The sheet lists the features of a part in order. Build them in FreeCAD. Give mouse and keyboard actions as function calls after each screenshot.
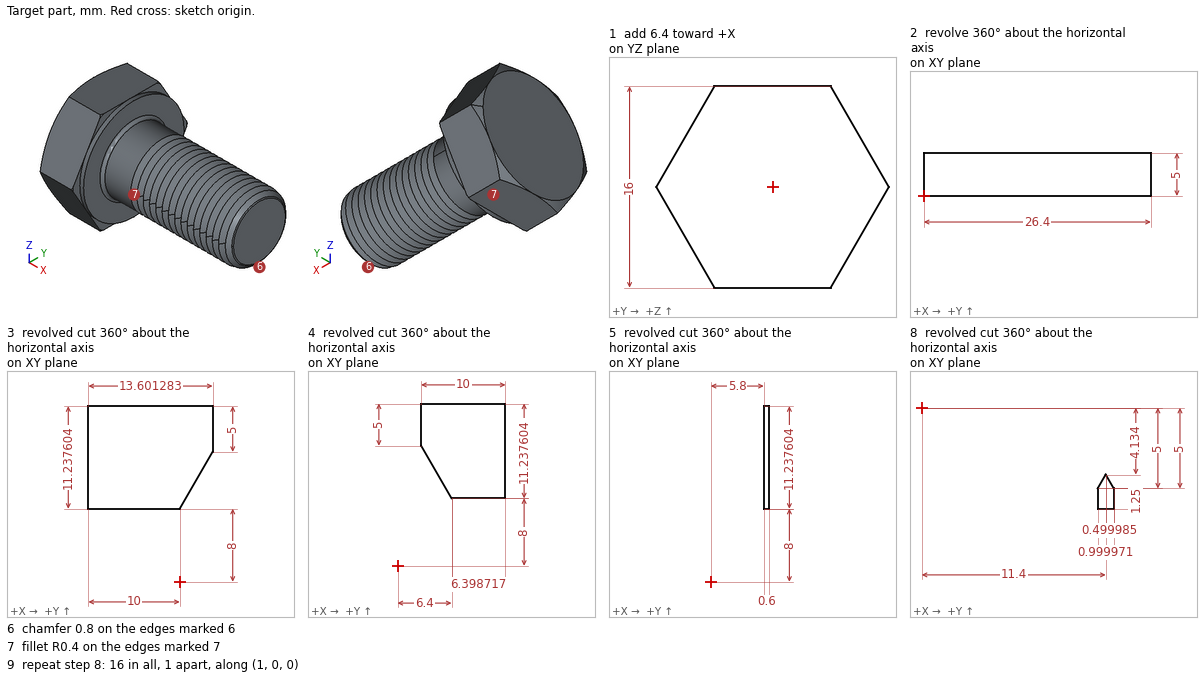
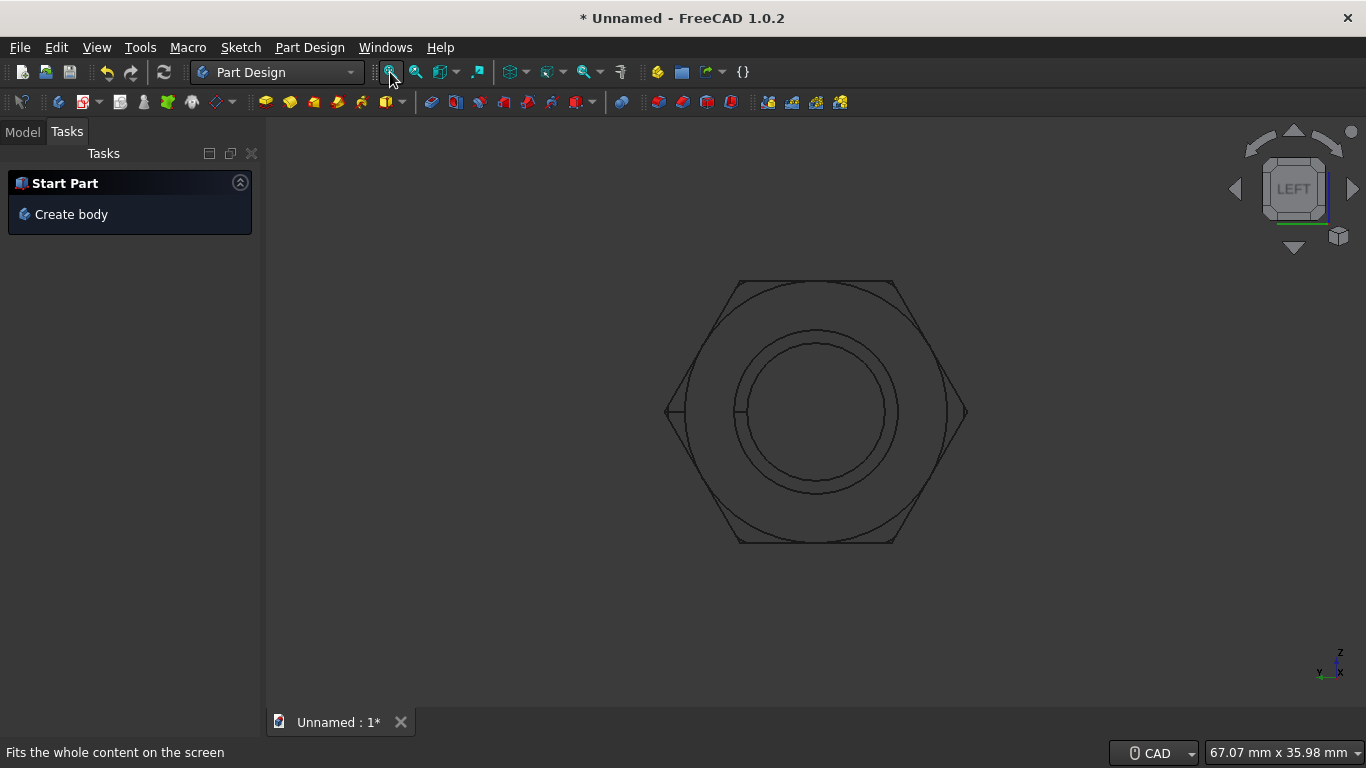
key(0)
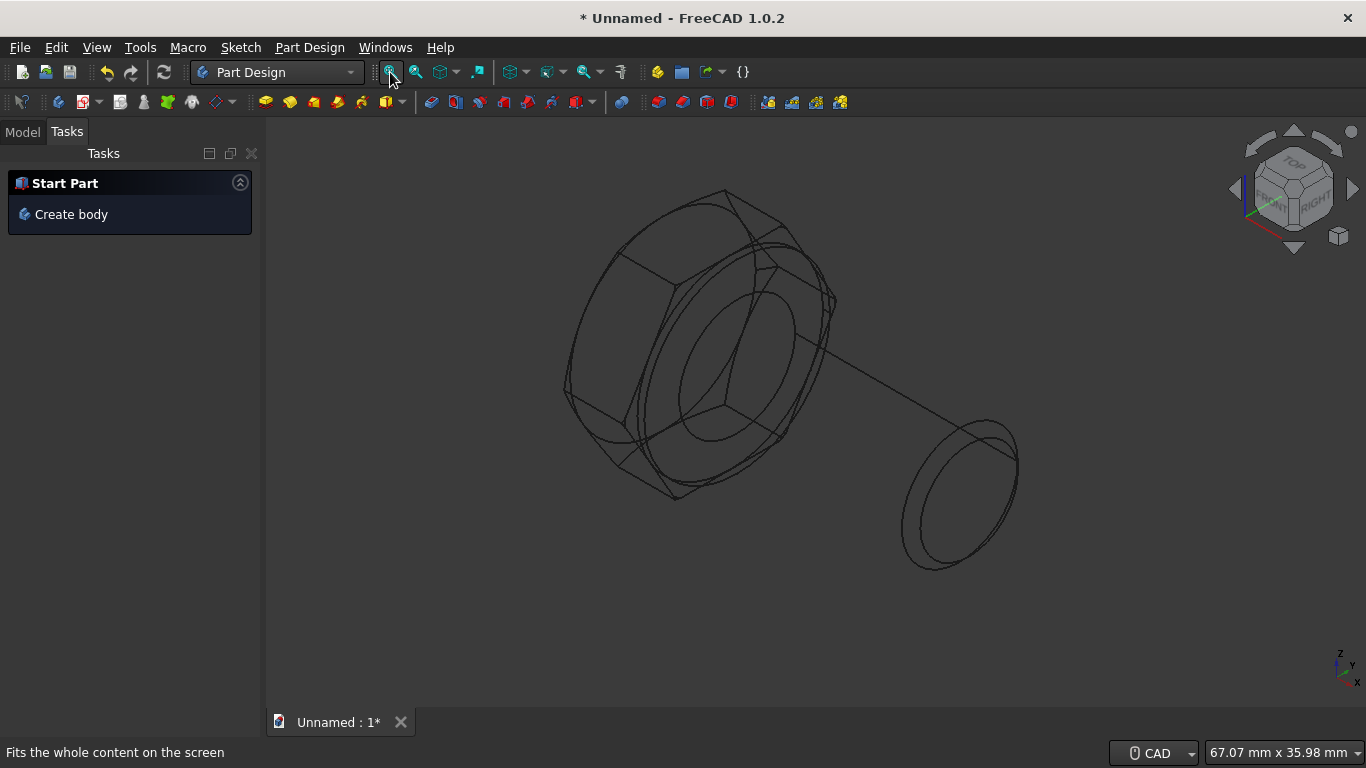
click(679, 399)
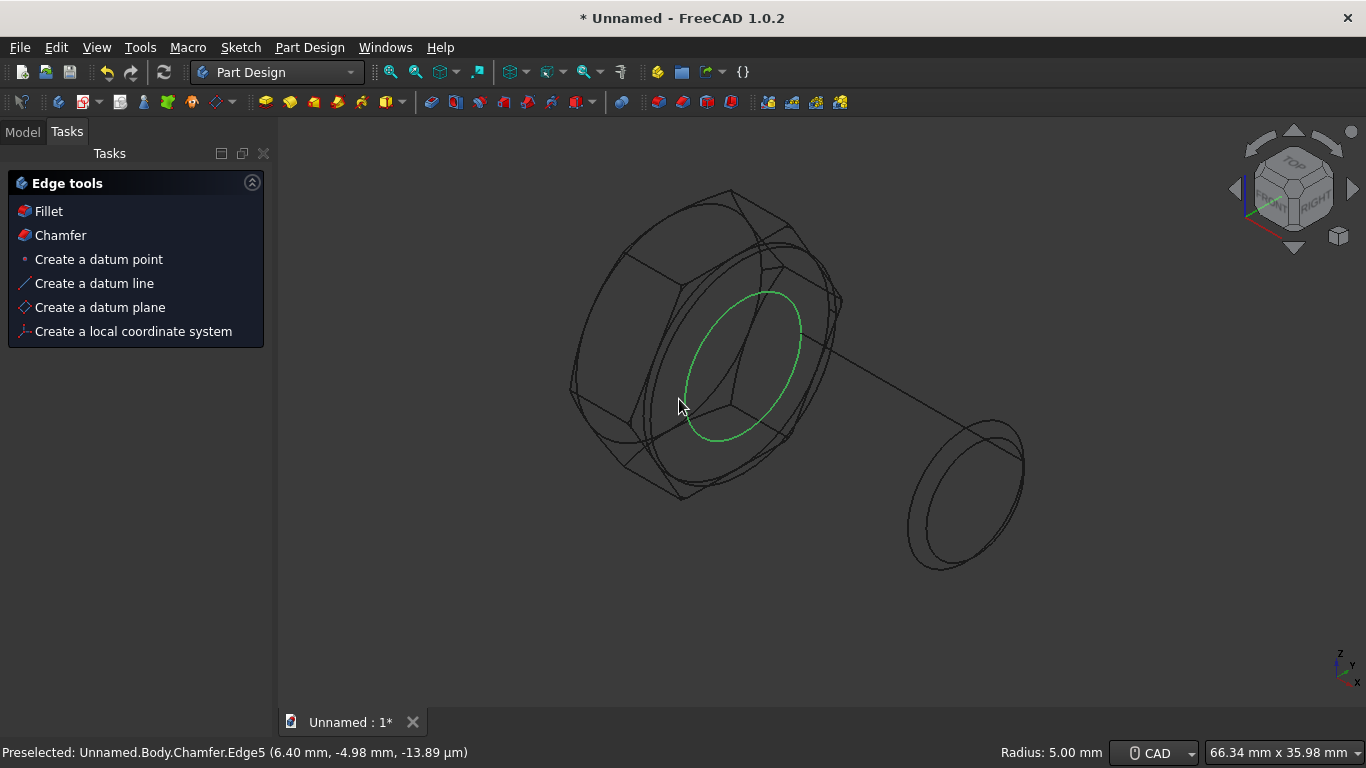
key(v)
key(1)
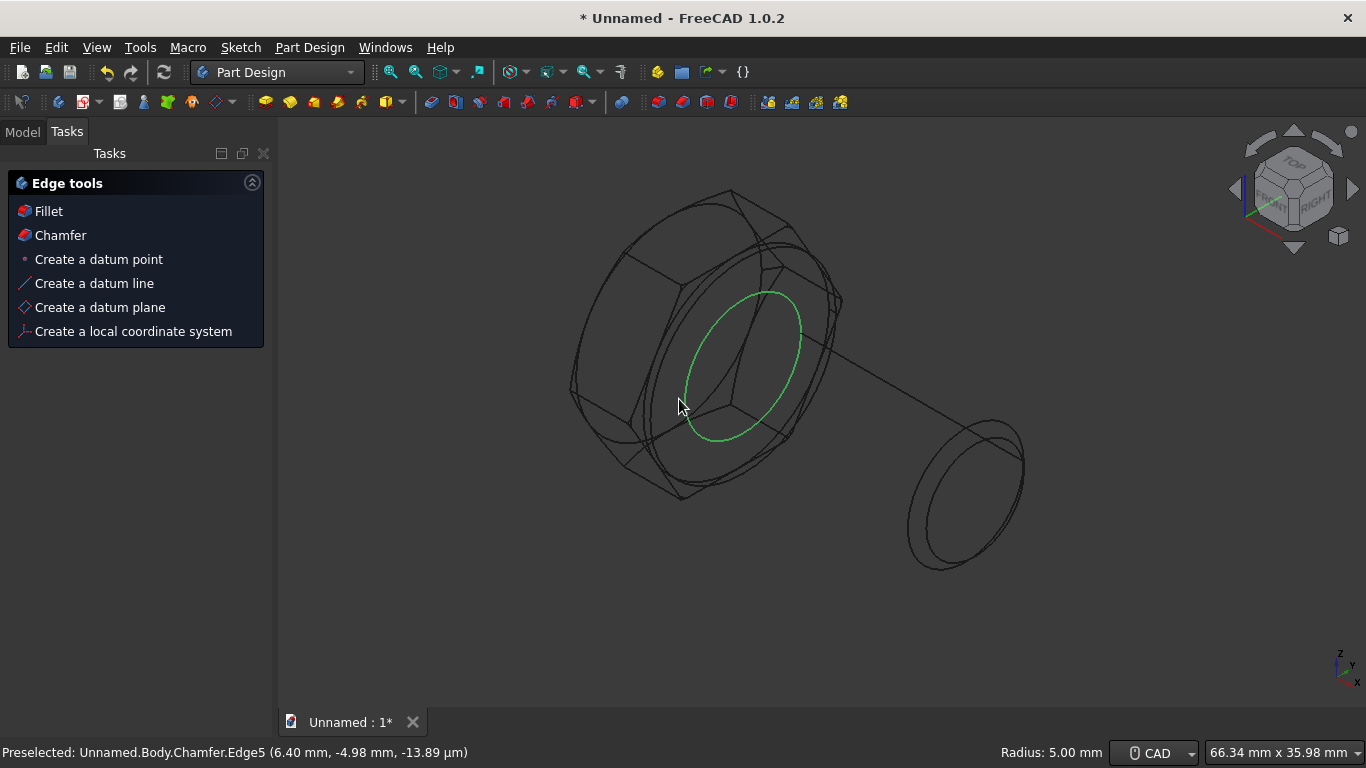
click(660, 102)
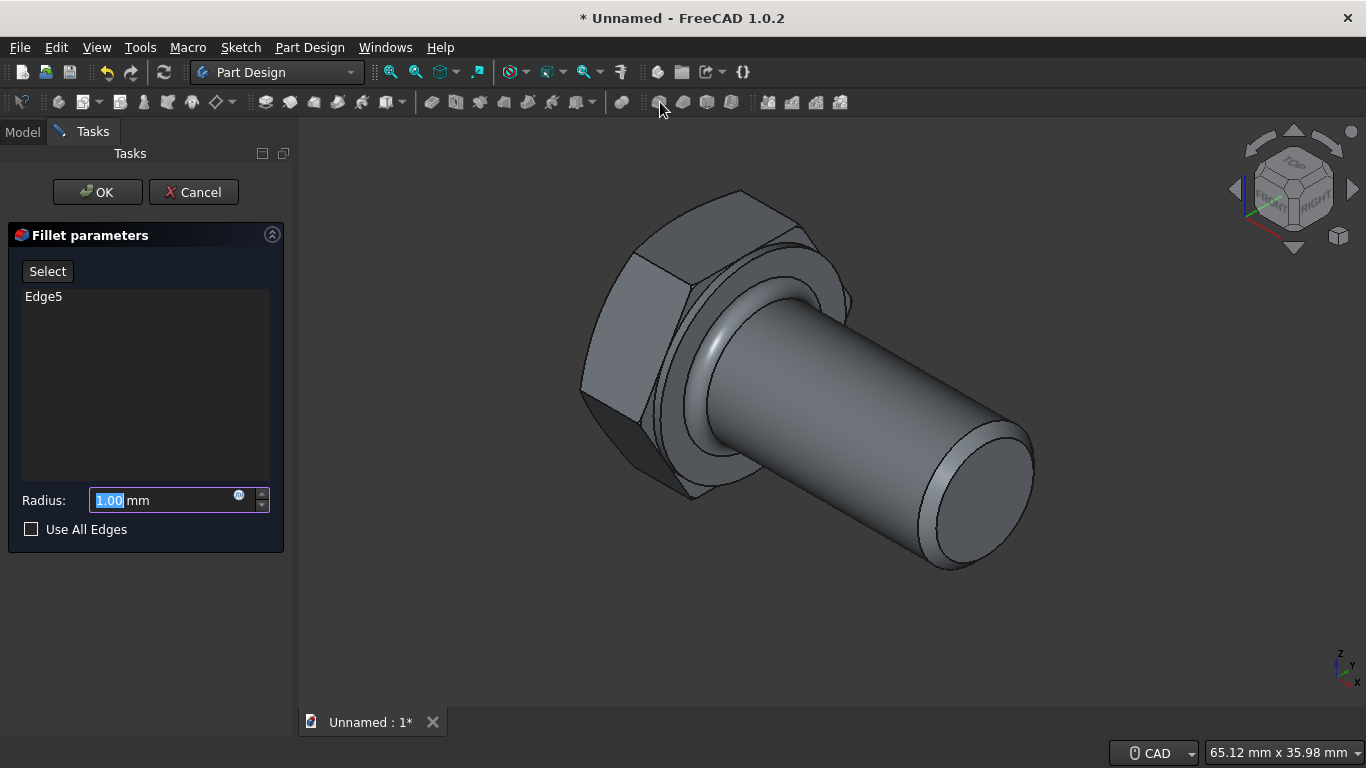
text(0.4)
key(Tab)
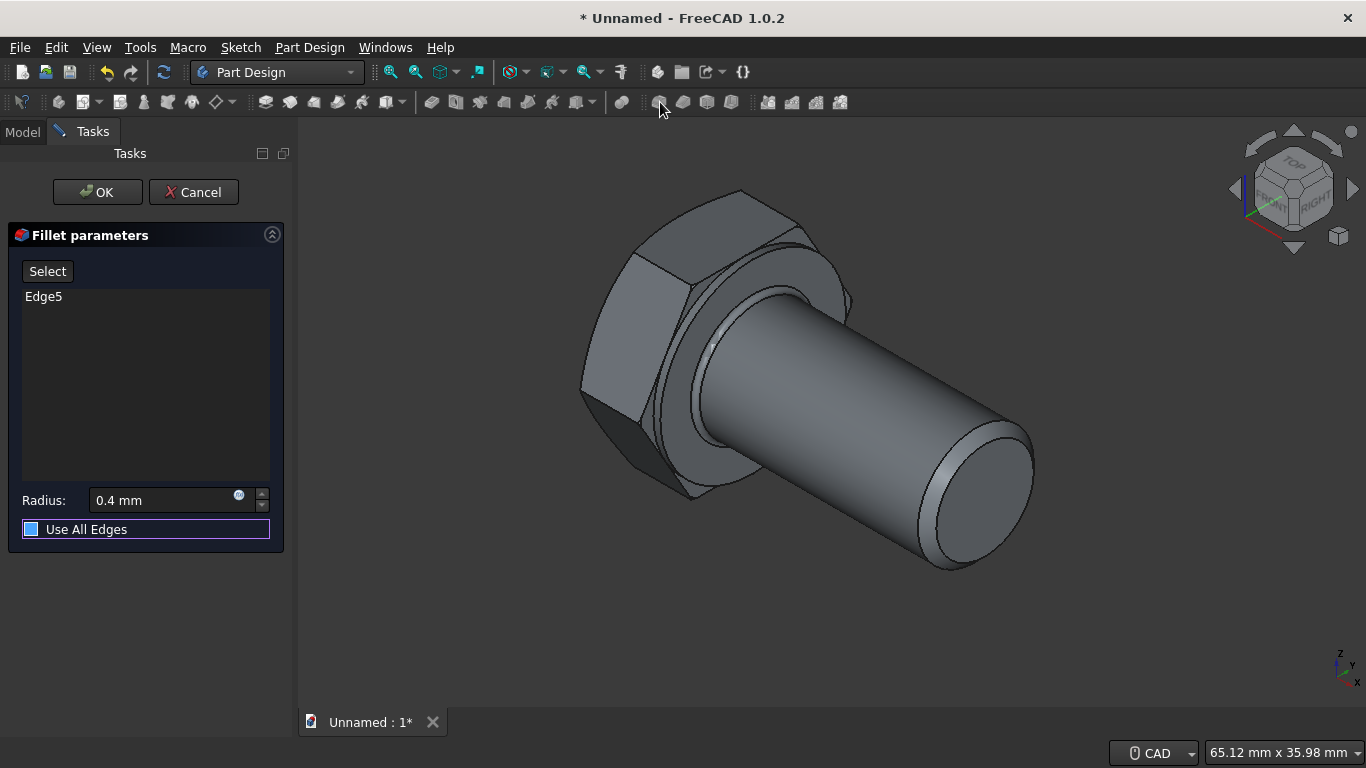
click(98, 192)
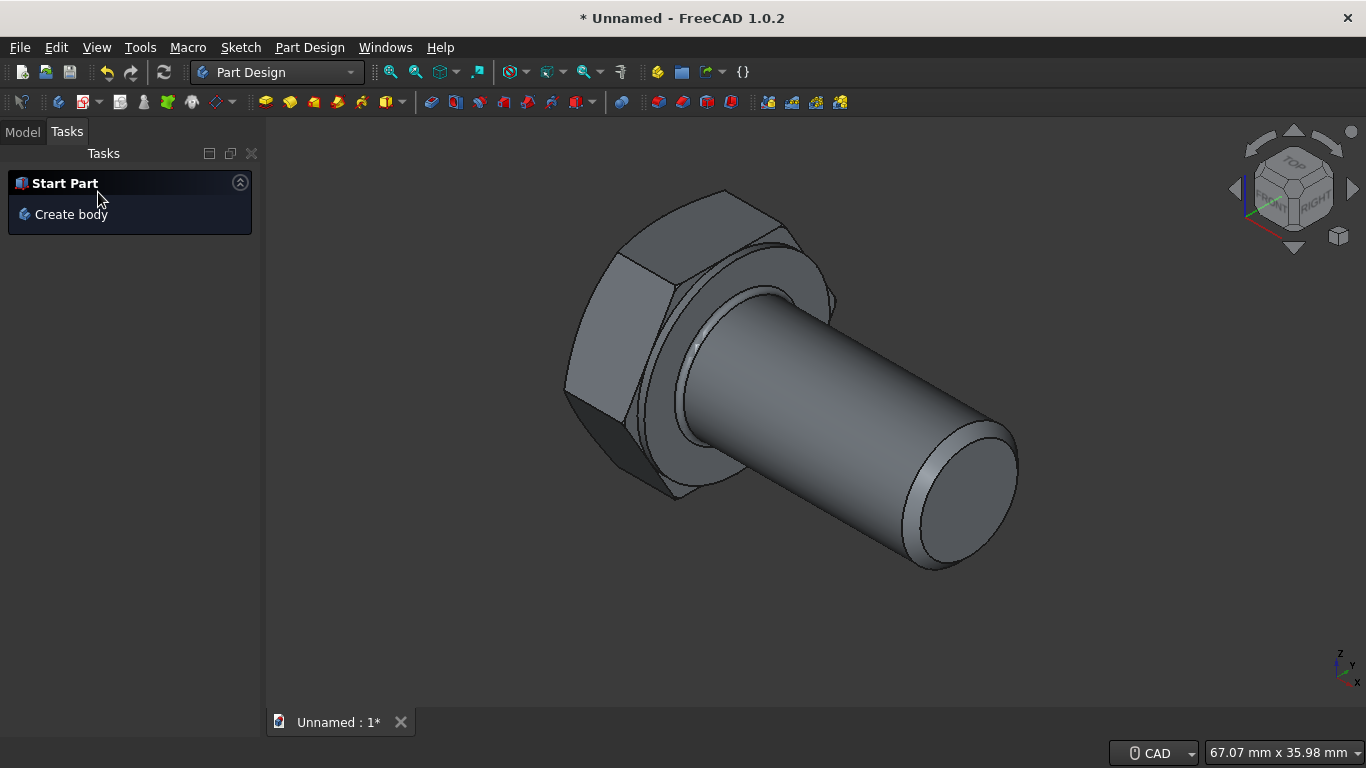
click(84, 102)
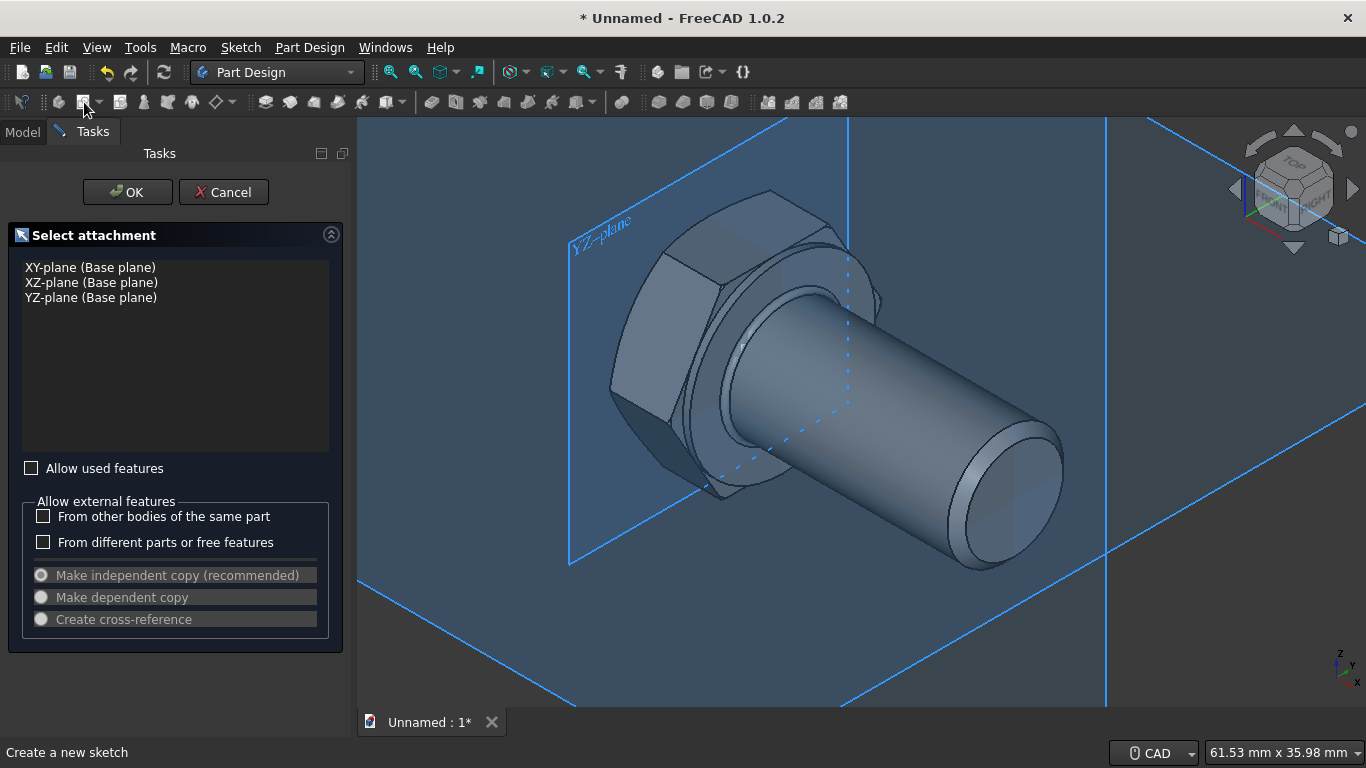
click(82, 268)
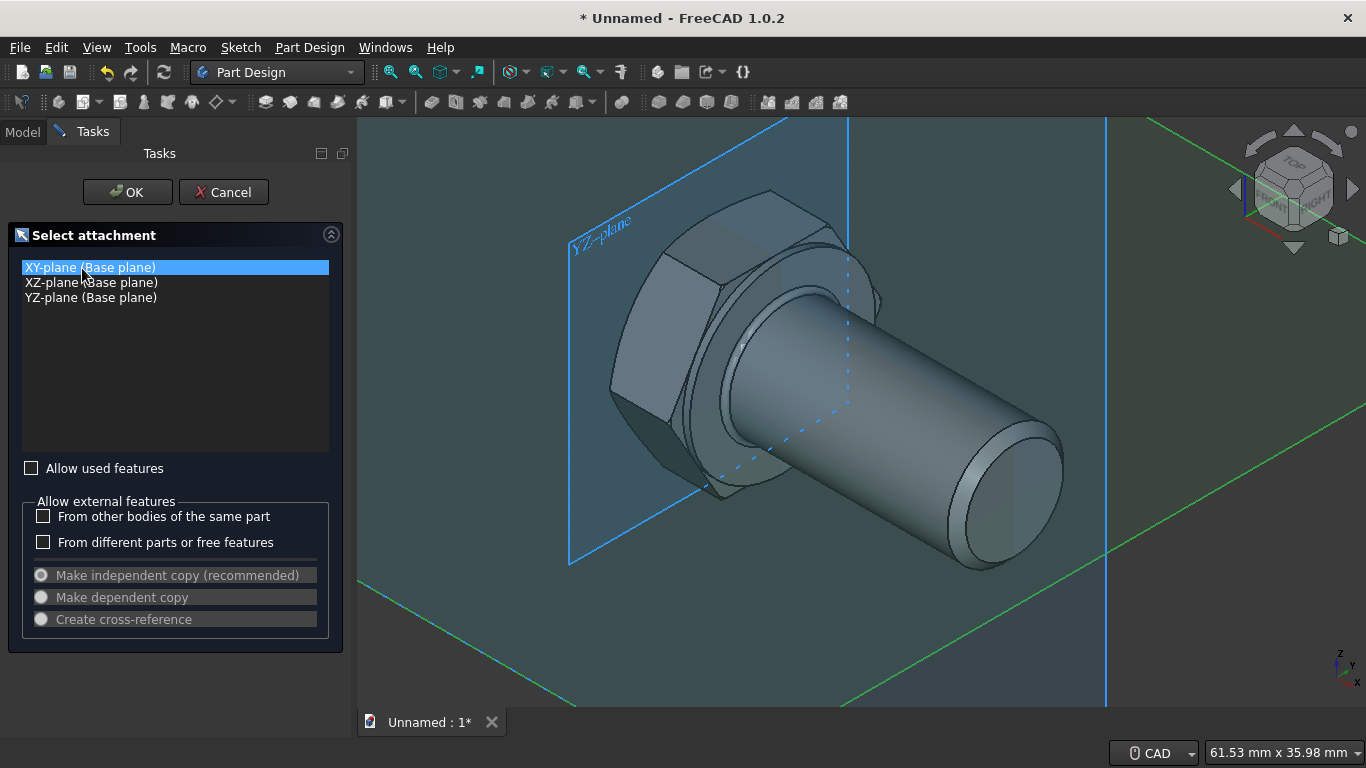
click(128, 192)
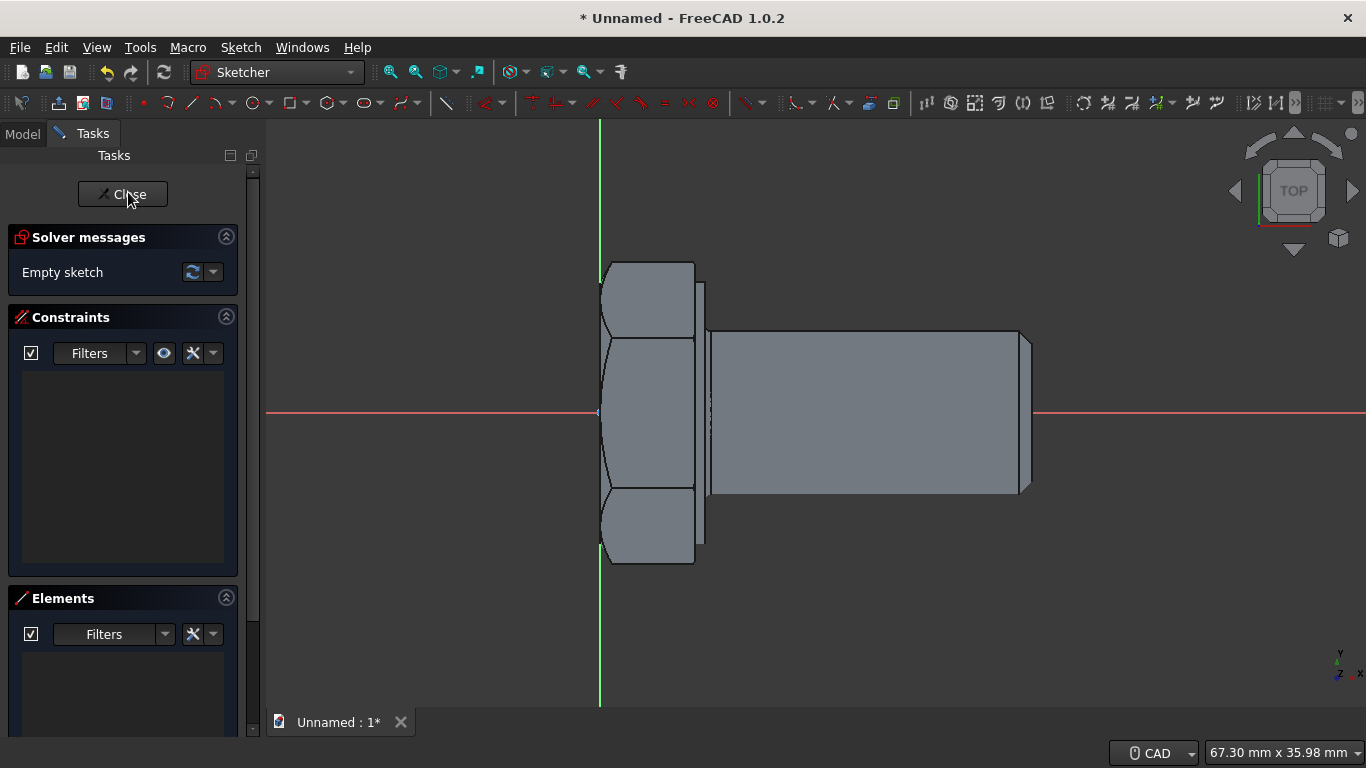
key(q)
key(s)